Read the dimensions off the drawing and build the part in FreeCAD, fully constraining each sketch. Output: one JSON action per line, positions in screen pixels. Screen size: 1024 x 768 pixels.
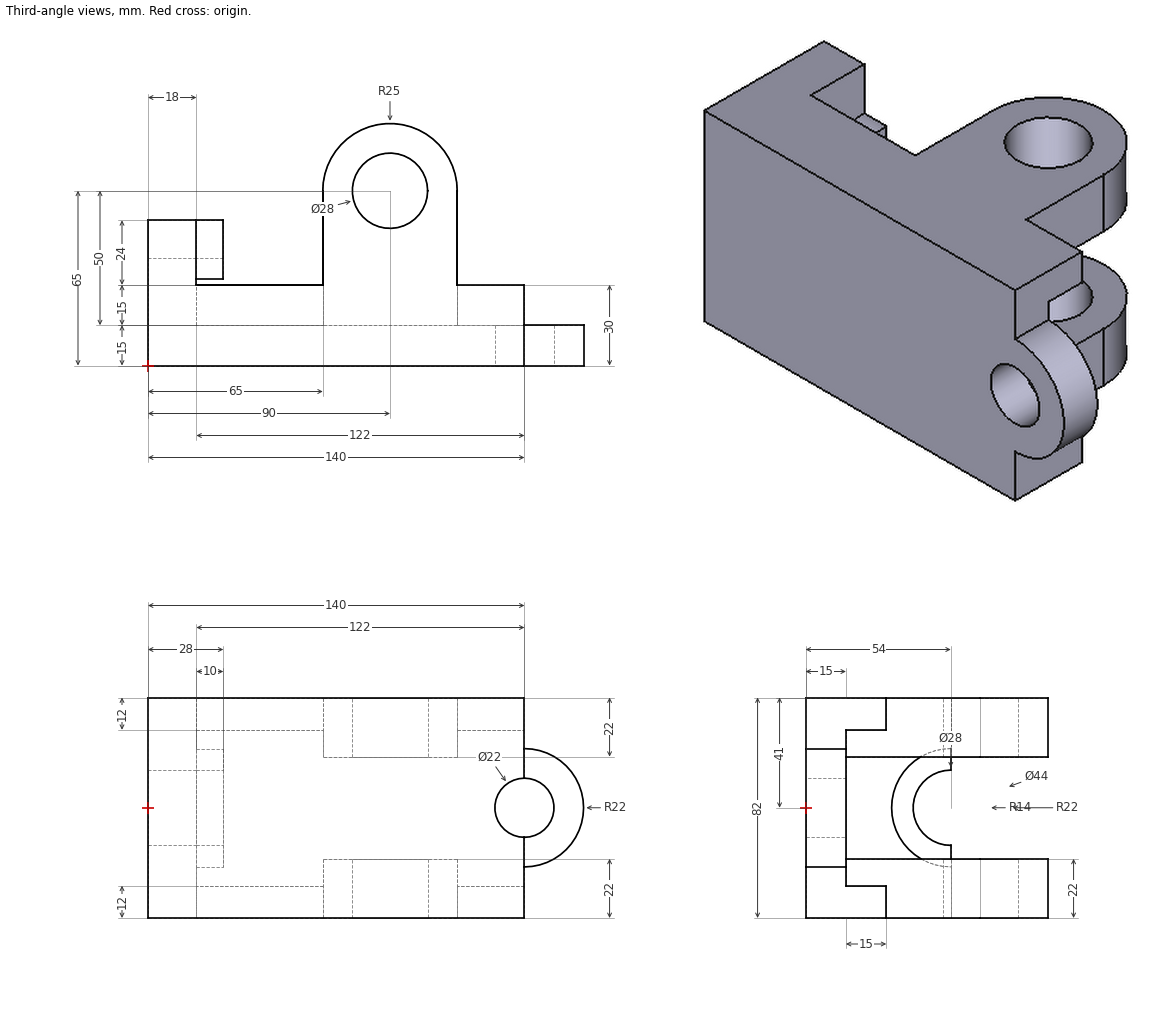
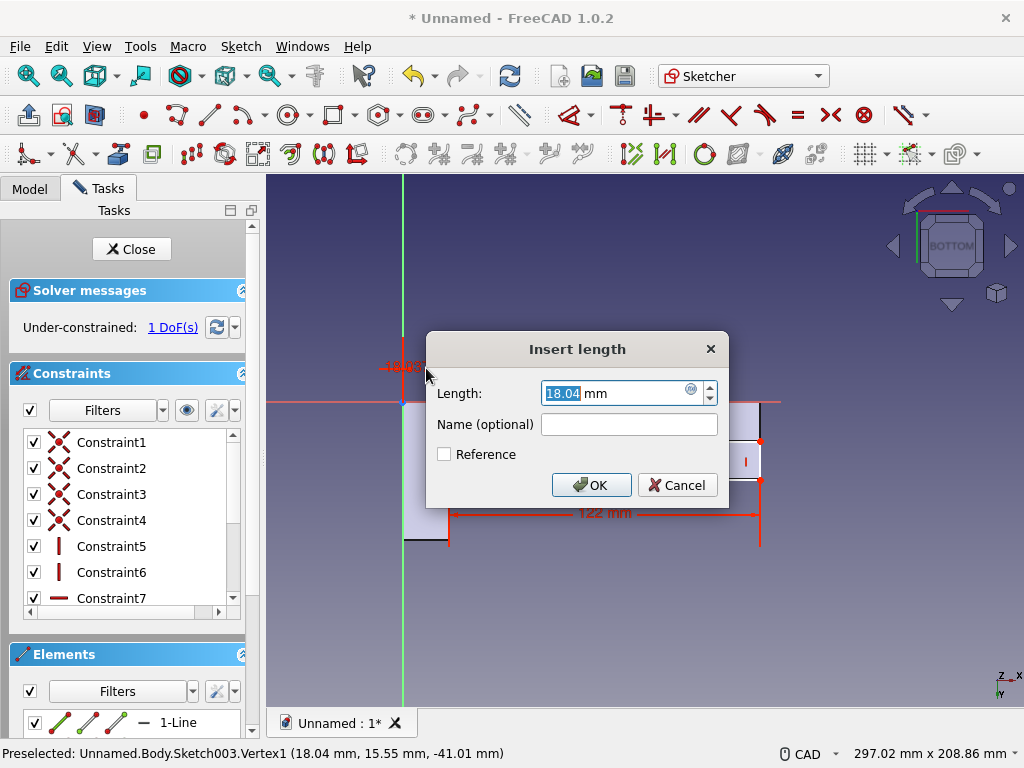
{"action": "type", "text": "18"}
{"action": "key", "text": "Return"}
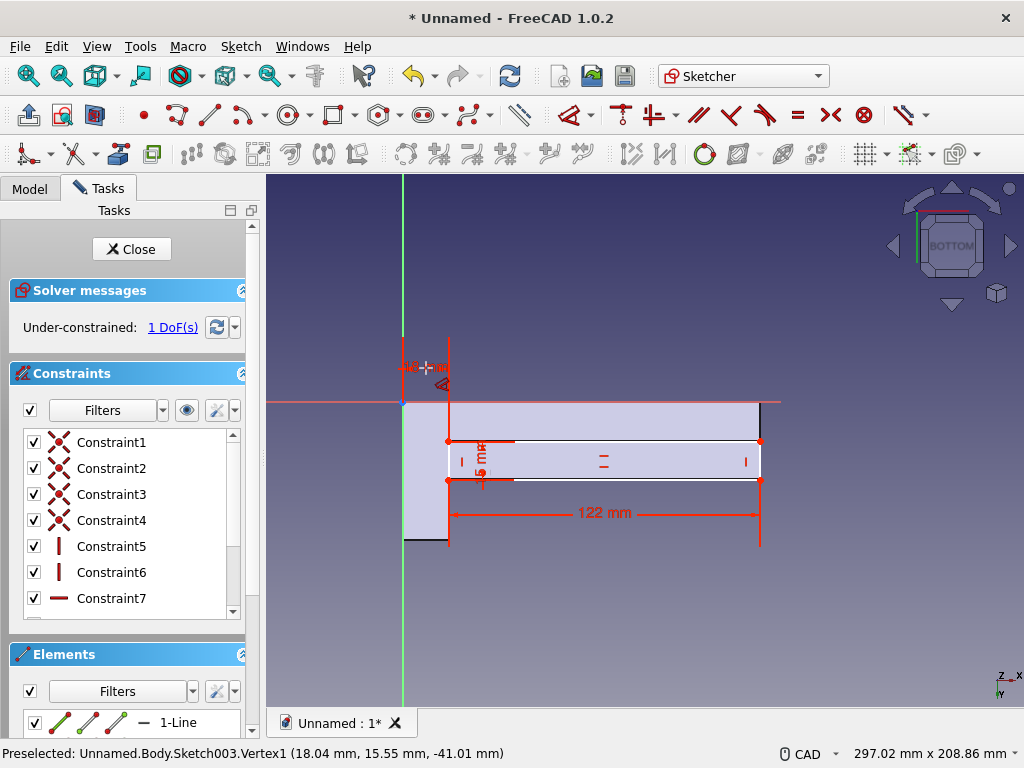
{"action": "left_click", "coordinate": [449, 442]}
{"action": "left_click", "coordinate": [369, 422]}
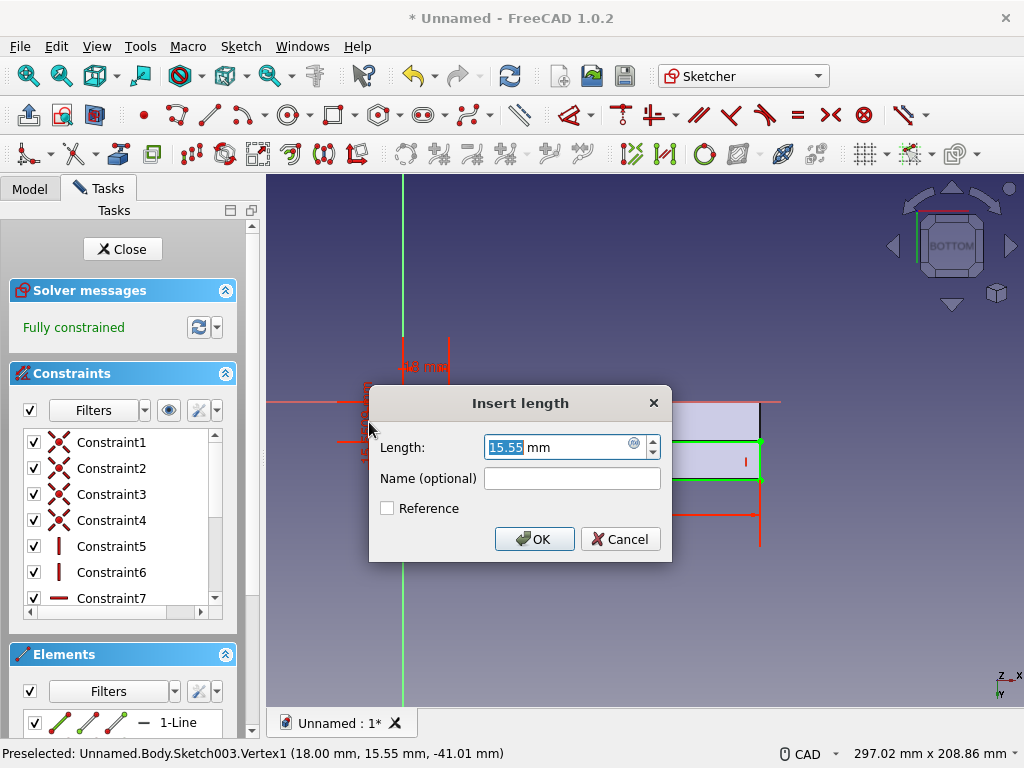
{"action": "type", "text": "15"}
{"action": "key", "text": "Return"}
{"action": "key", "text": "Escape"}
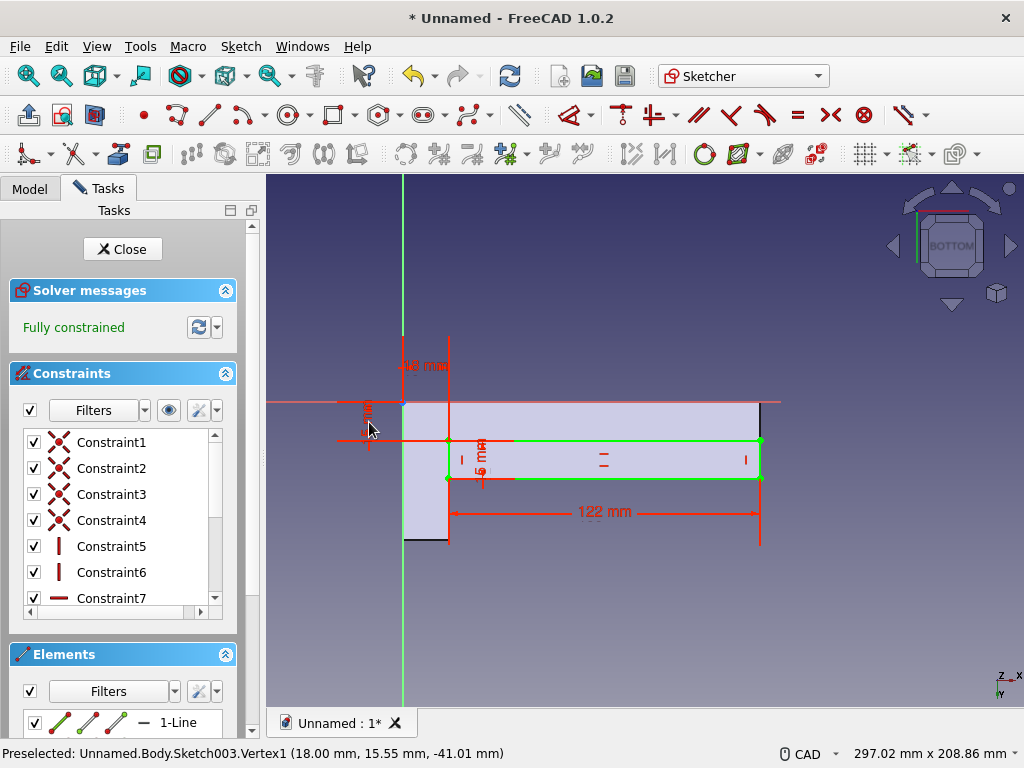
{"action": "left_click", "coordinate": [123, 249]}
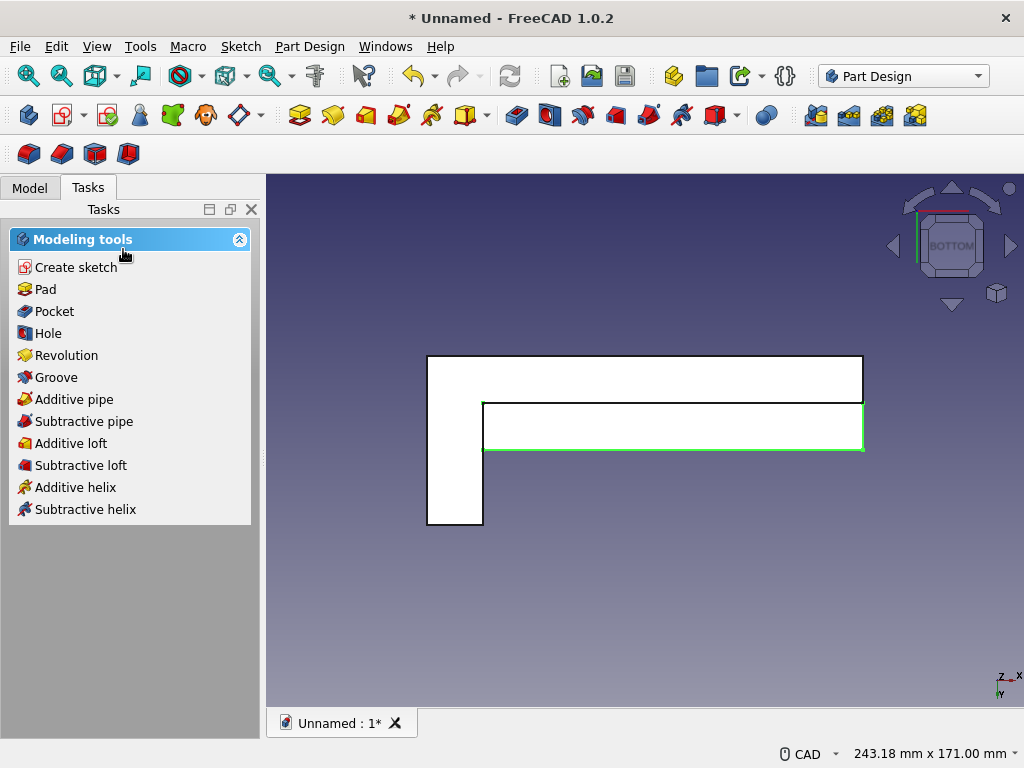
{"action": "left_click", "coordinate": [300, 116]}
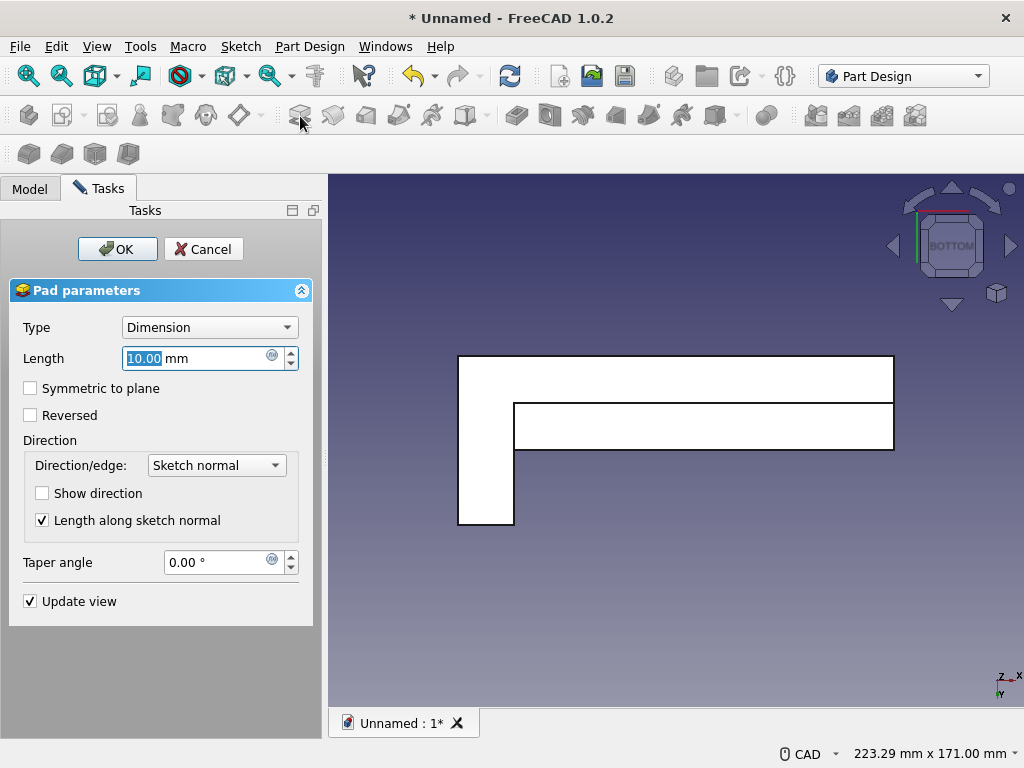
{"action": "type", "text": "12"}
{"action": "key", "text": "Tab"}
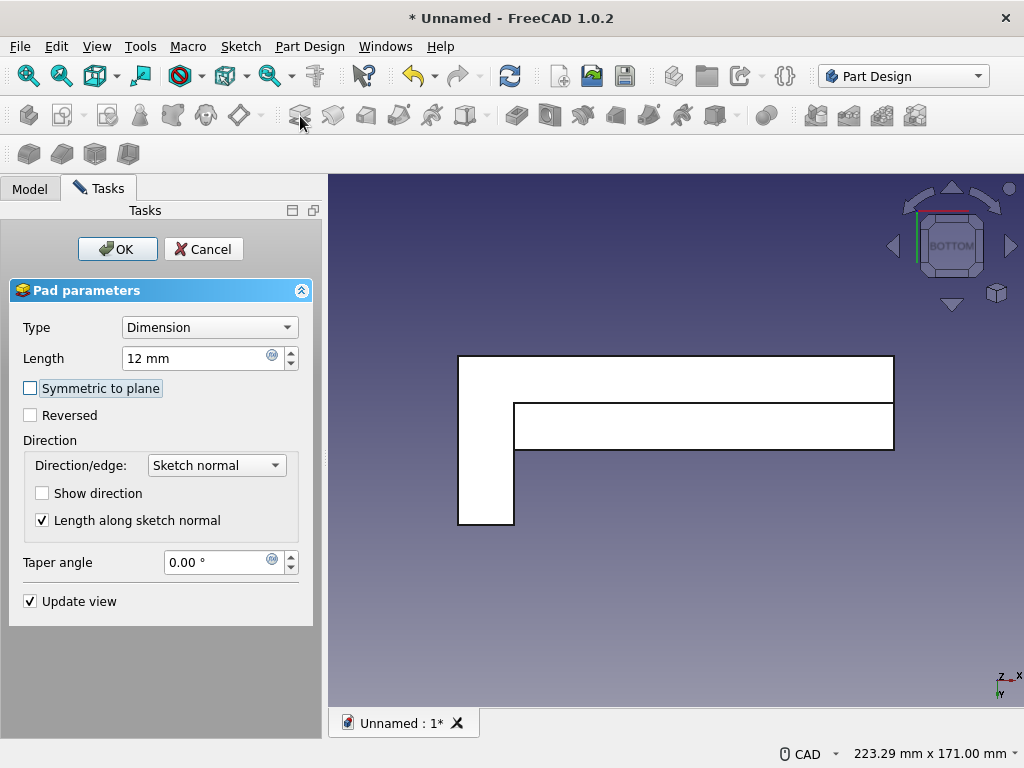
{"action": "left_click", "coordinate": [31, 415]}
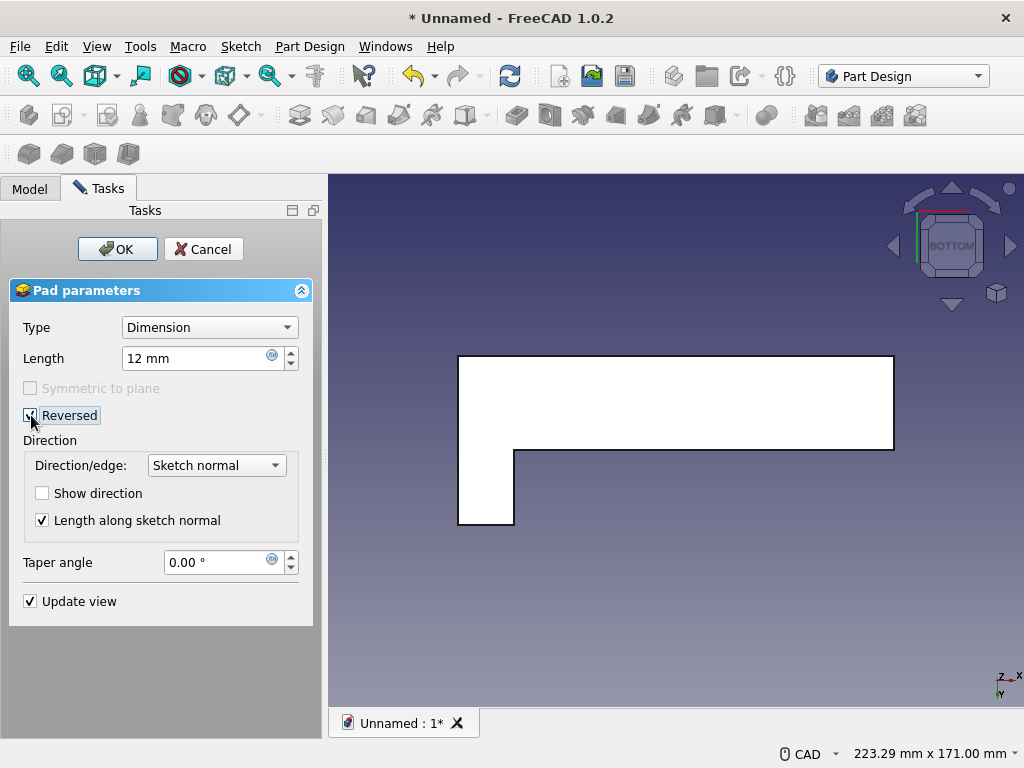
{"action": "left_click", "coordinate": [118, 249]}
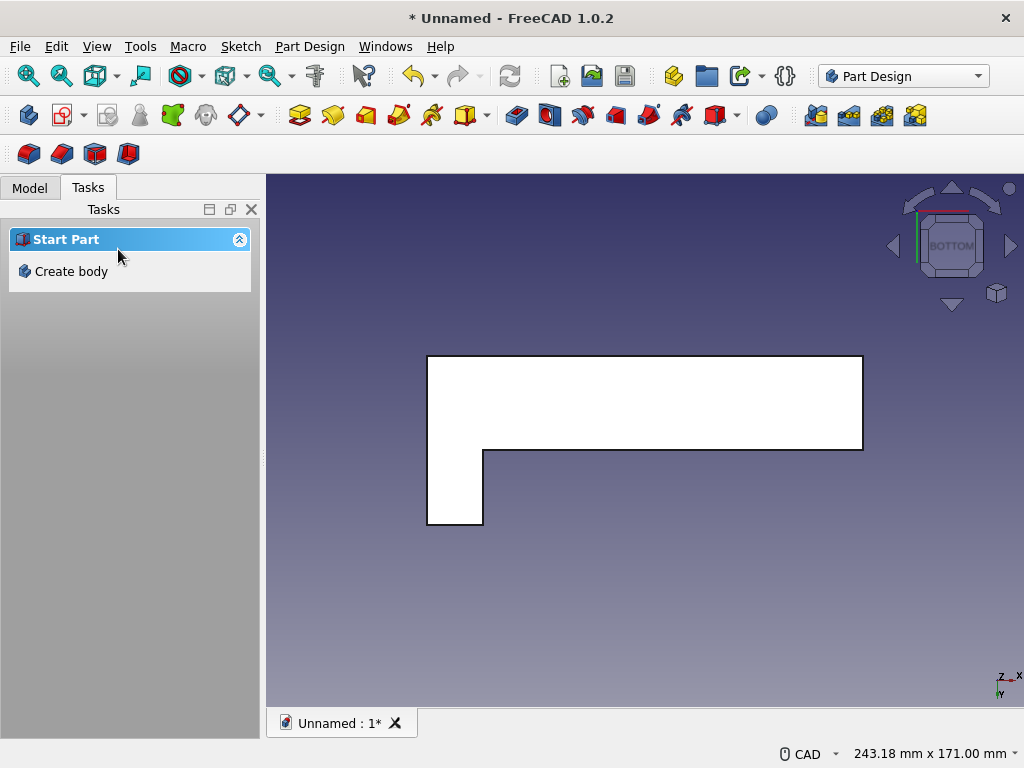
{"action": "key", "text": "0"}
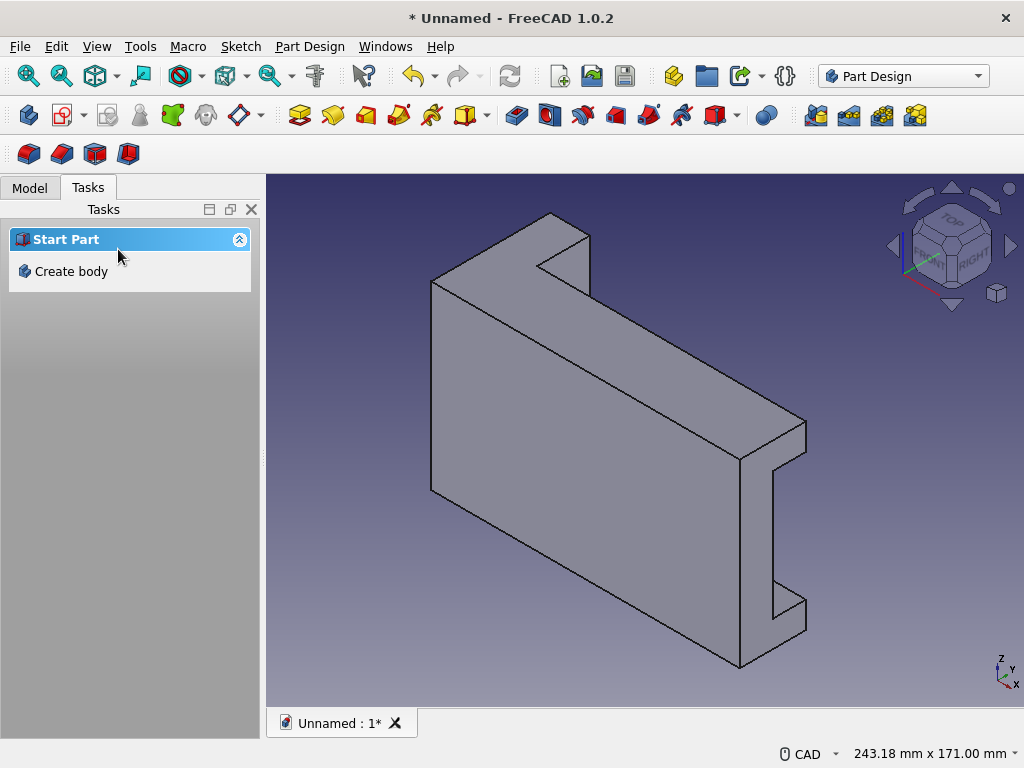
{"action": "left_click", "coordinate": [699, 406]}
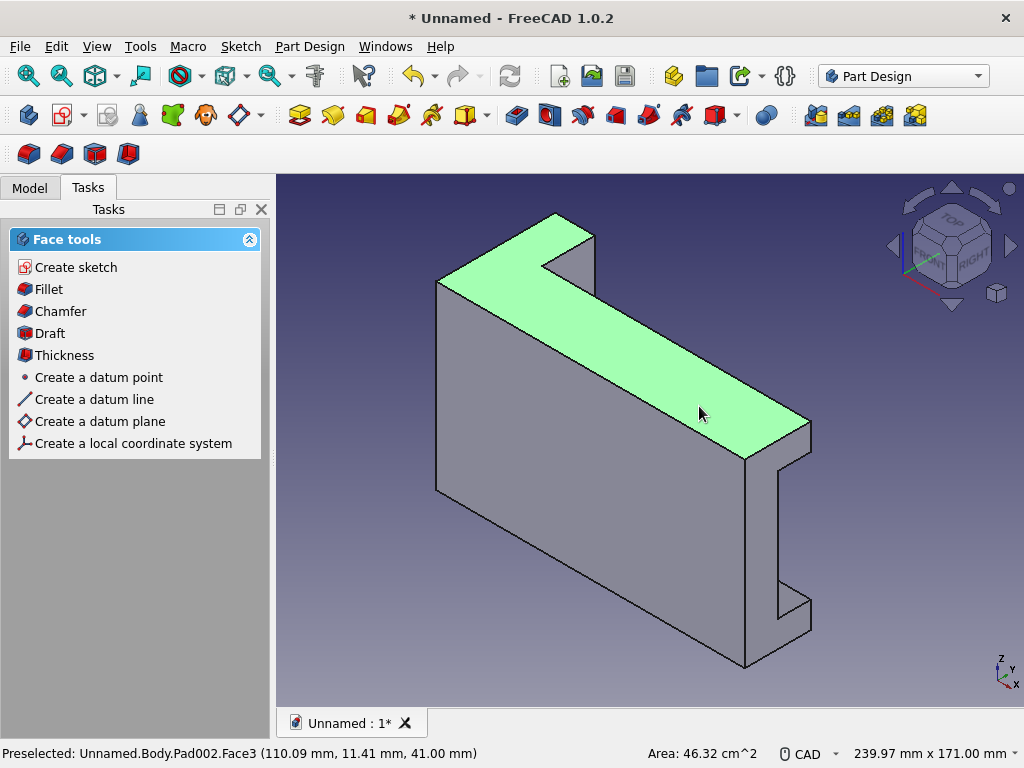
{"action": "left_click", "coordinate": [62, 116]}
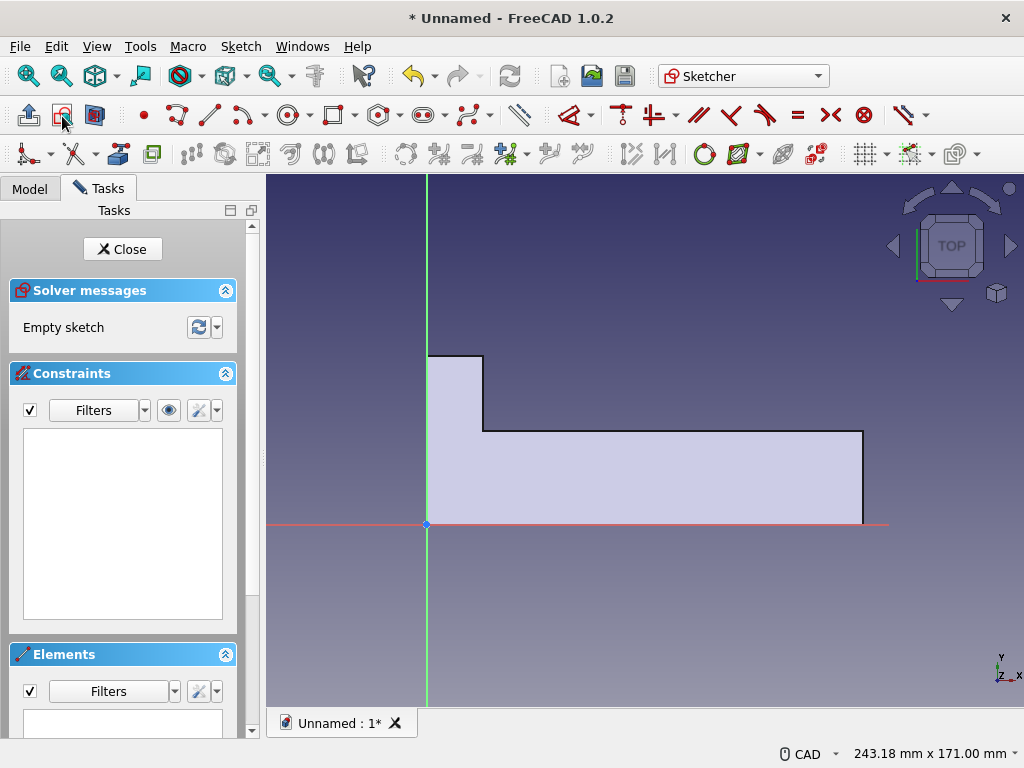
{"action": "left_click", "coordinate": [177, 116]}